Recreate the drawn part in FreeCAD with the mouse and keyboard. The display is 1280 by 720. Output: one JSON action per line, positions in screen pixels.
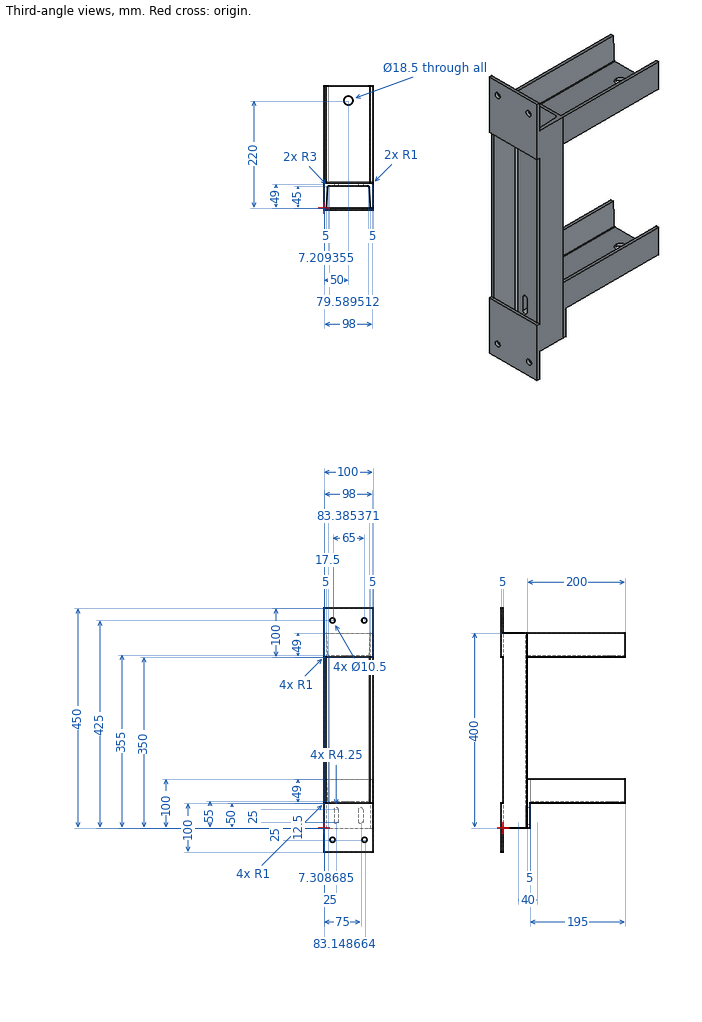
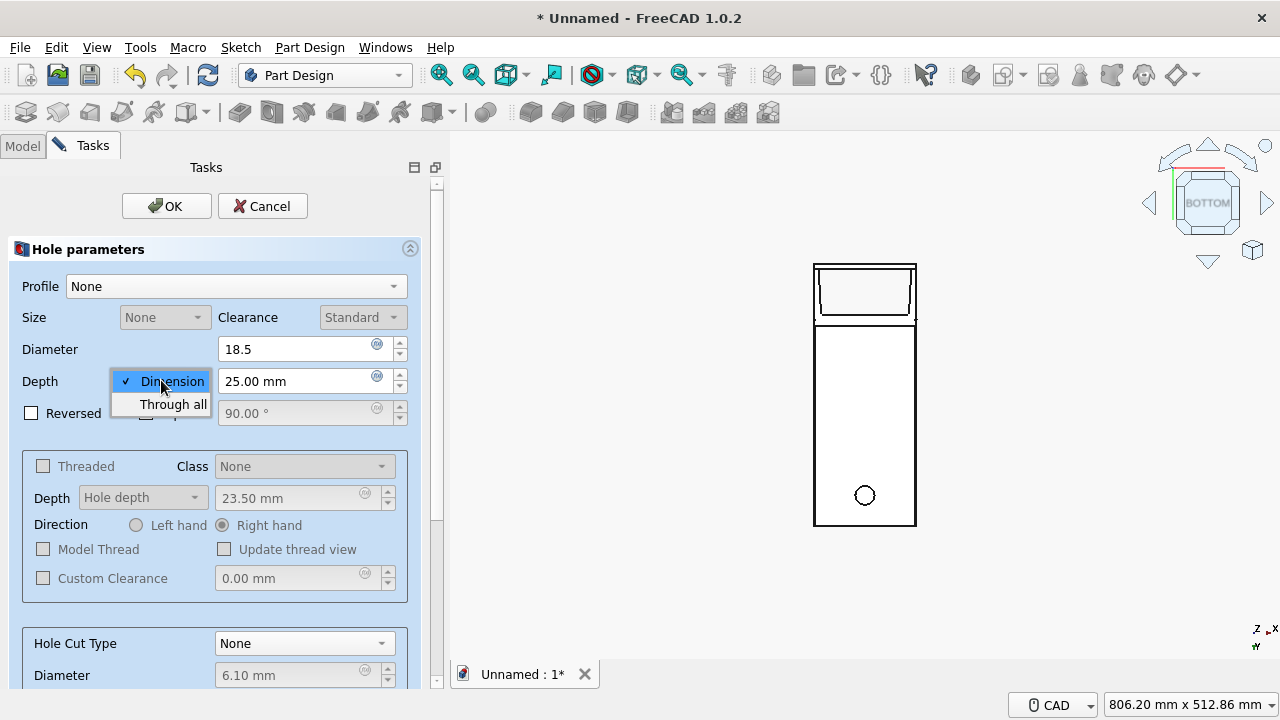
{"action": "left_click", "coordinate": [160, 404]}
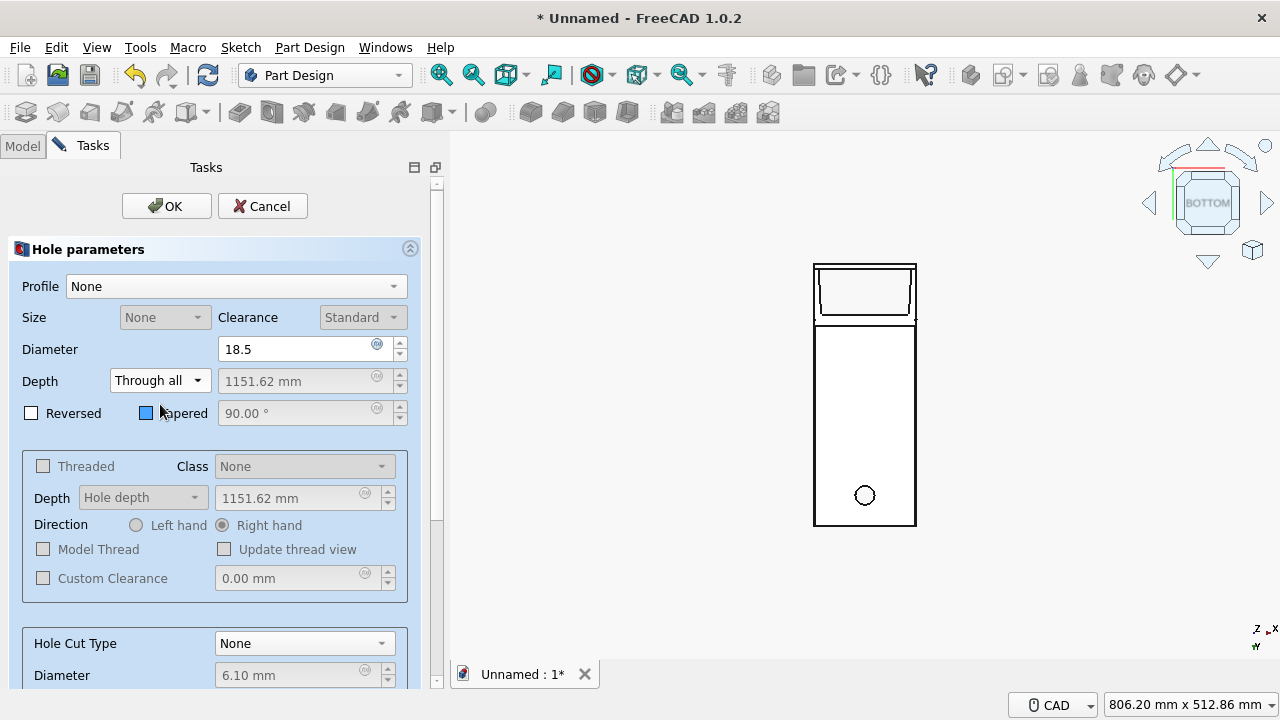
{"action": "left_click", "coordinate": [167, 206]}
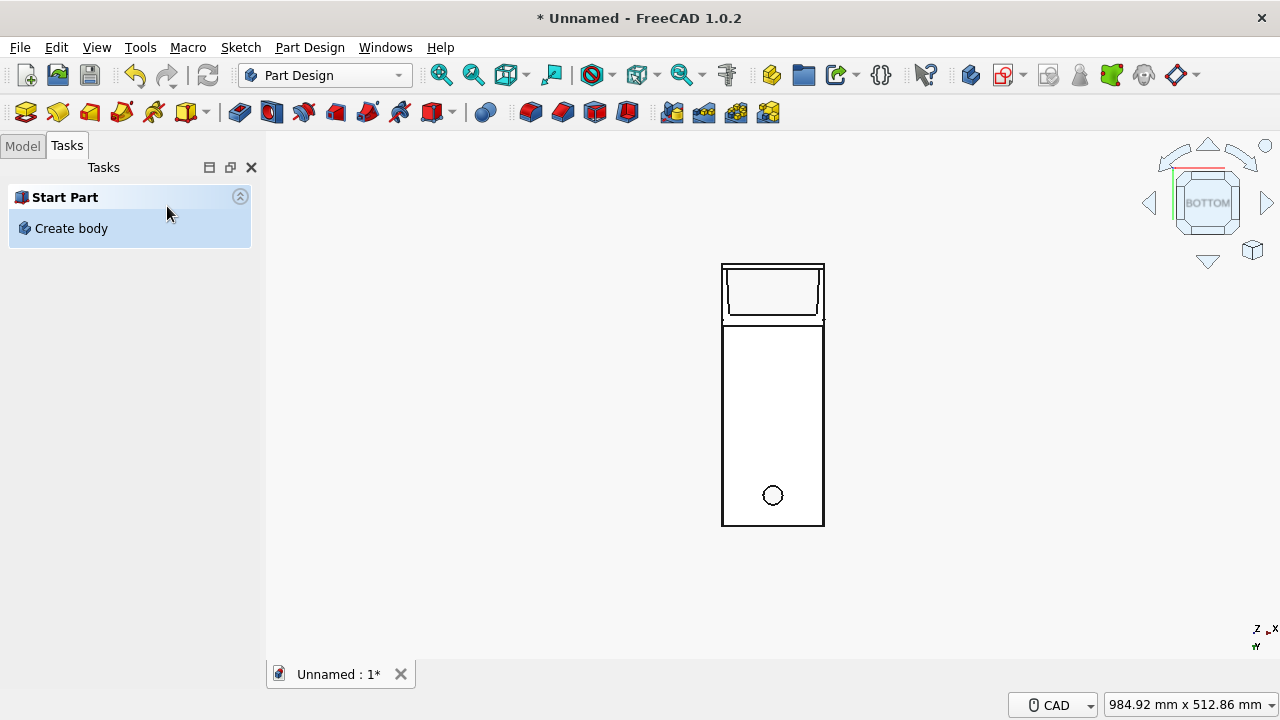
{"action": "key", "text": "0"}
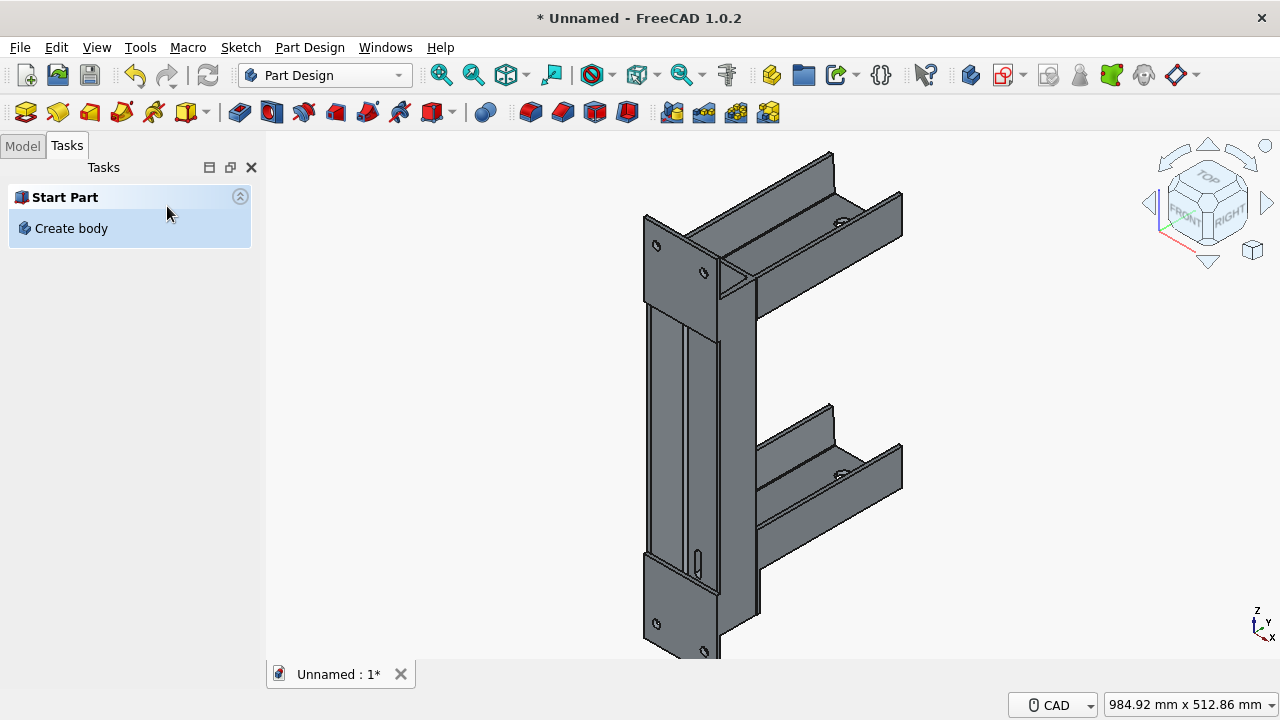
{"action": "left_click", "coordinate": [442, 76]}